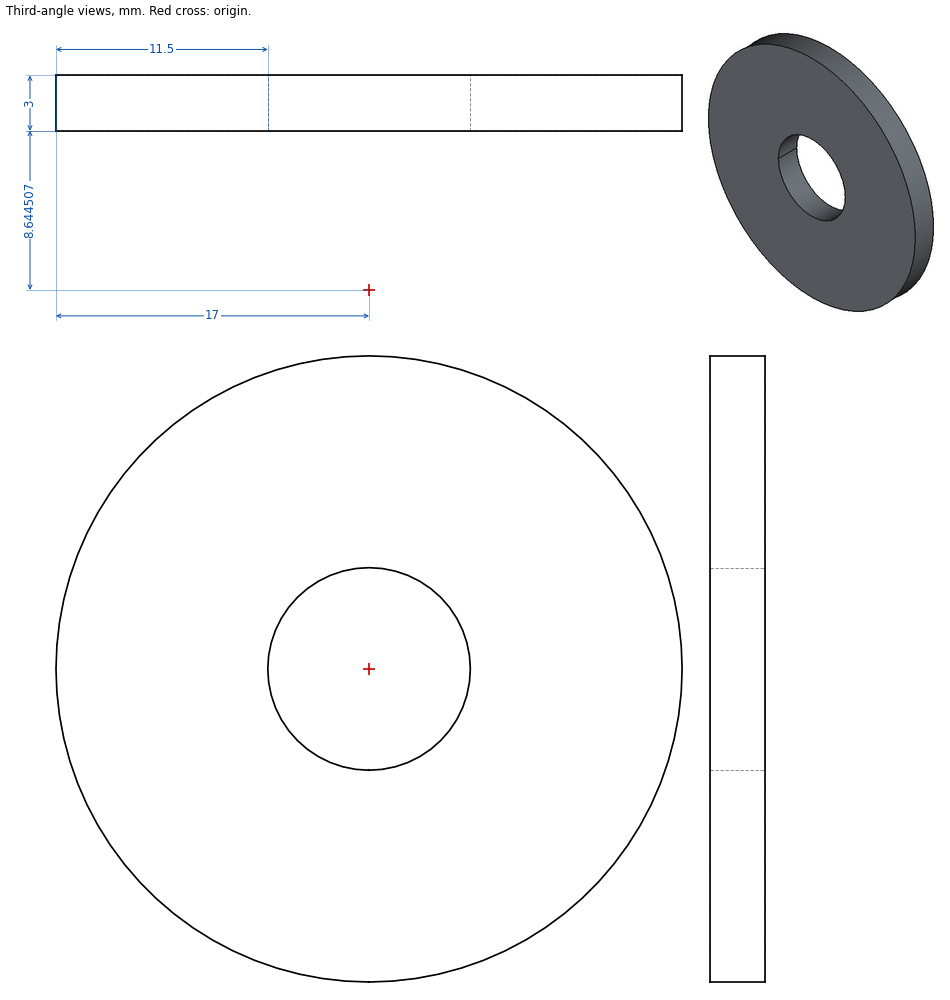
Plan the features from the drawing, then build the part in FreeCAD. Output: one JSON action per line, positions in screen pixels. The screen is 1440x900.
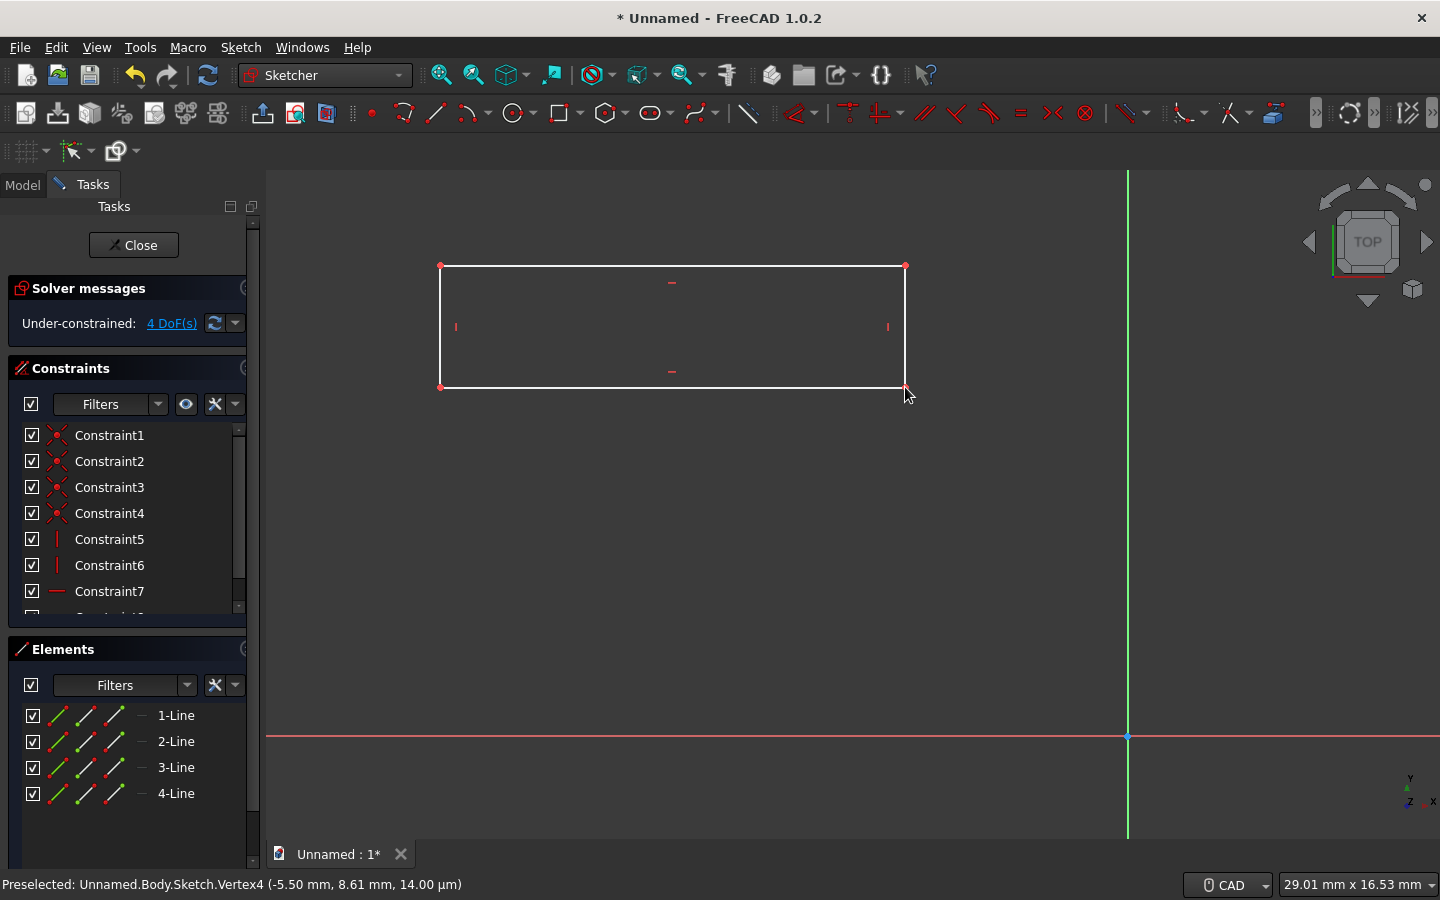
{"action": "left_click", "coordinate": [794, 114]}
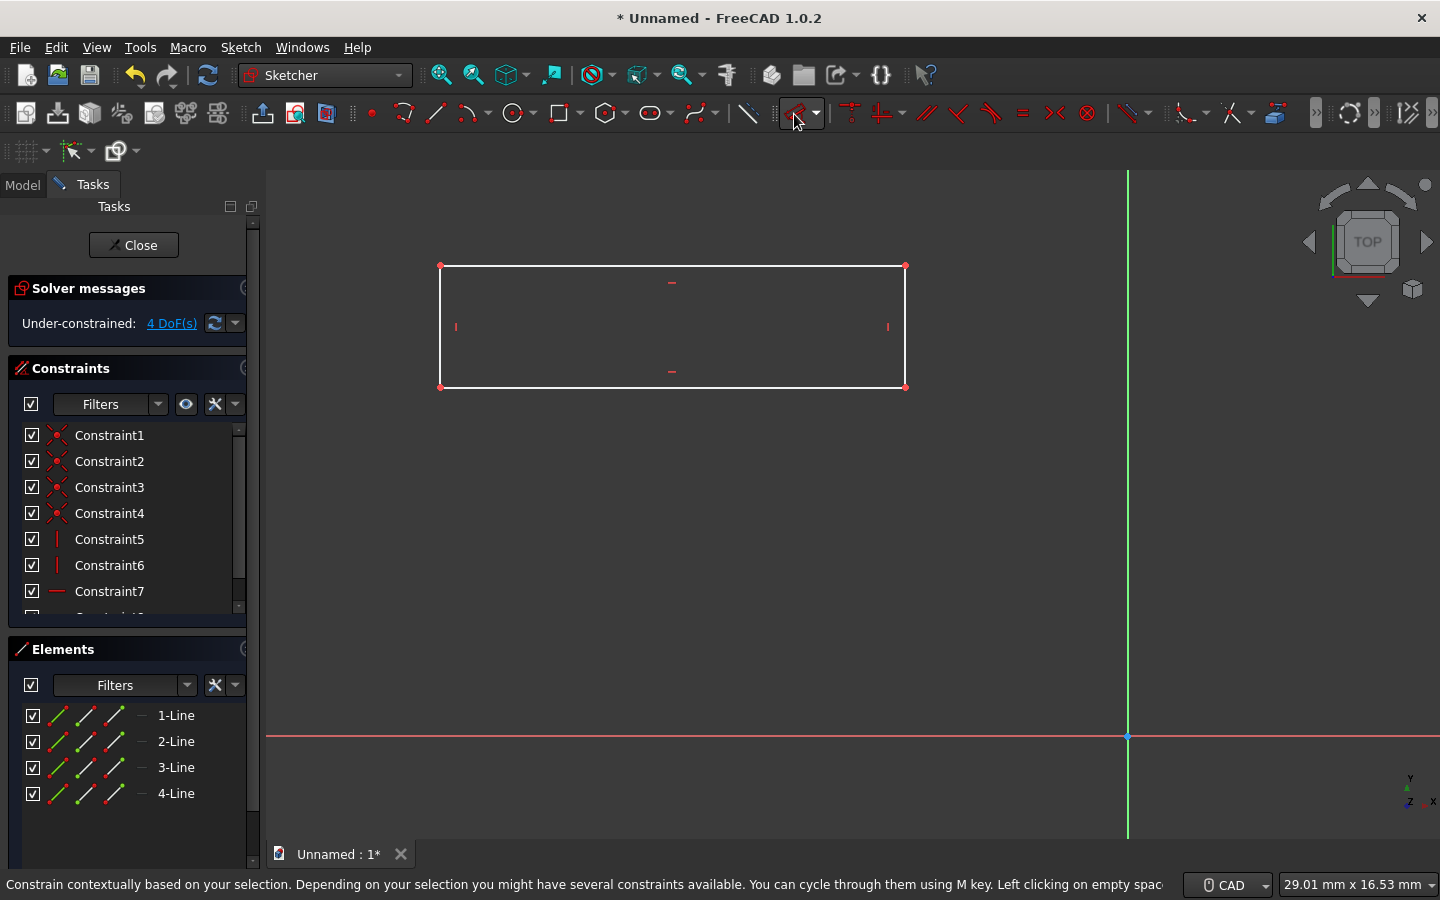
{"action": "left_click", "coordinate": [440, 303]}
{"action": "left_click", "coordinate": [406, 327]}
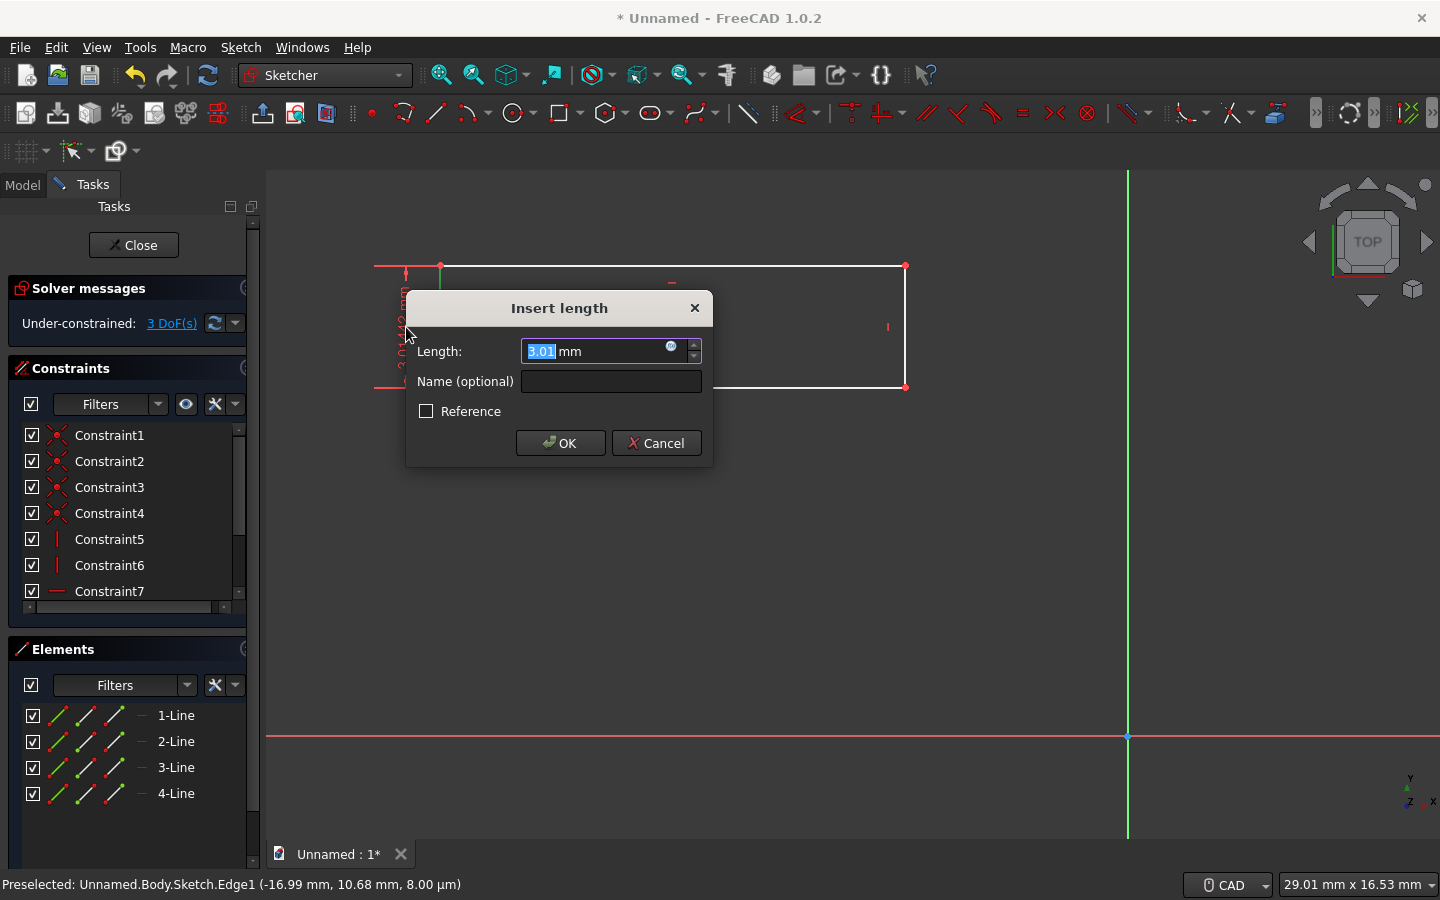
{"action": "type", "text": "3"}
{"action": "key", "text": "Return"}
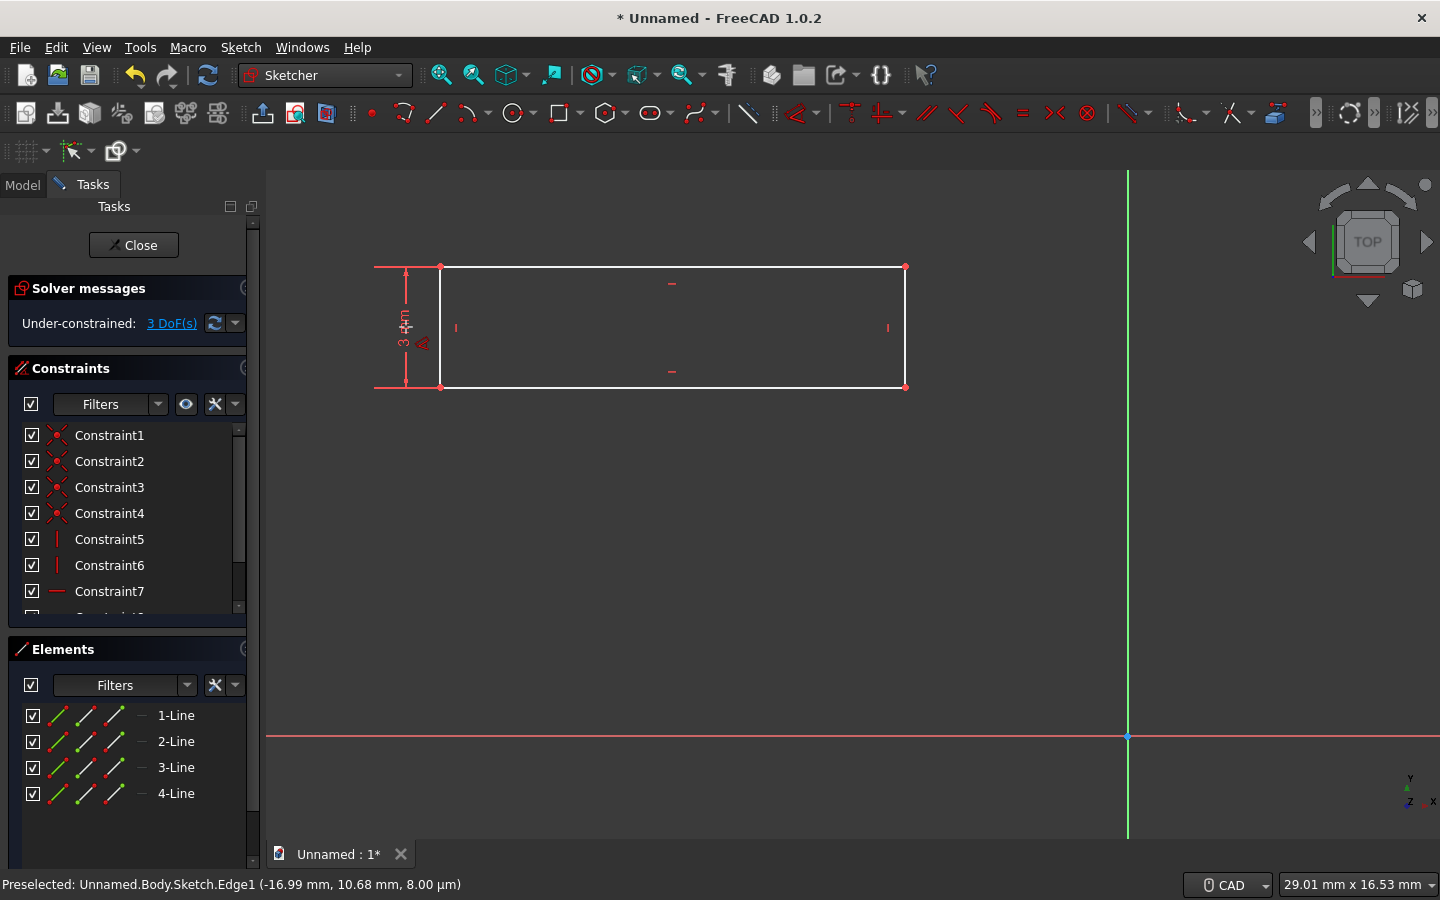
{"action": "left_click", "coordinate": [440, 267]}
{"action": "left_click", "coordinate": [784, 770]}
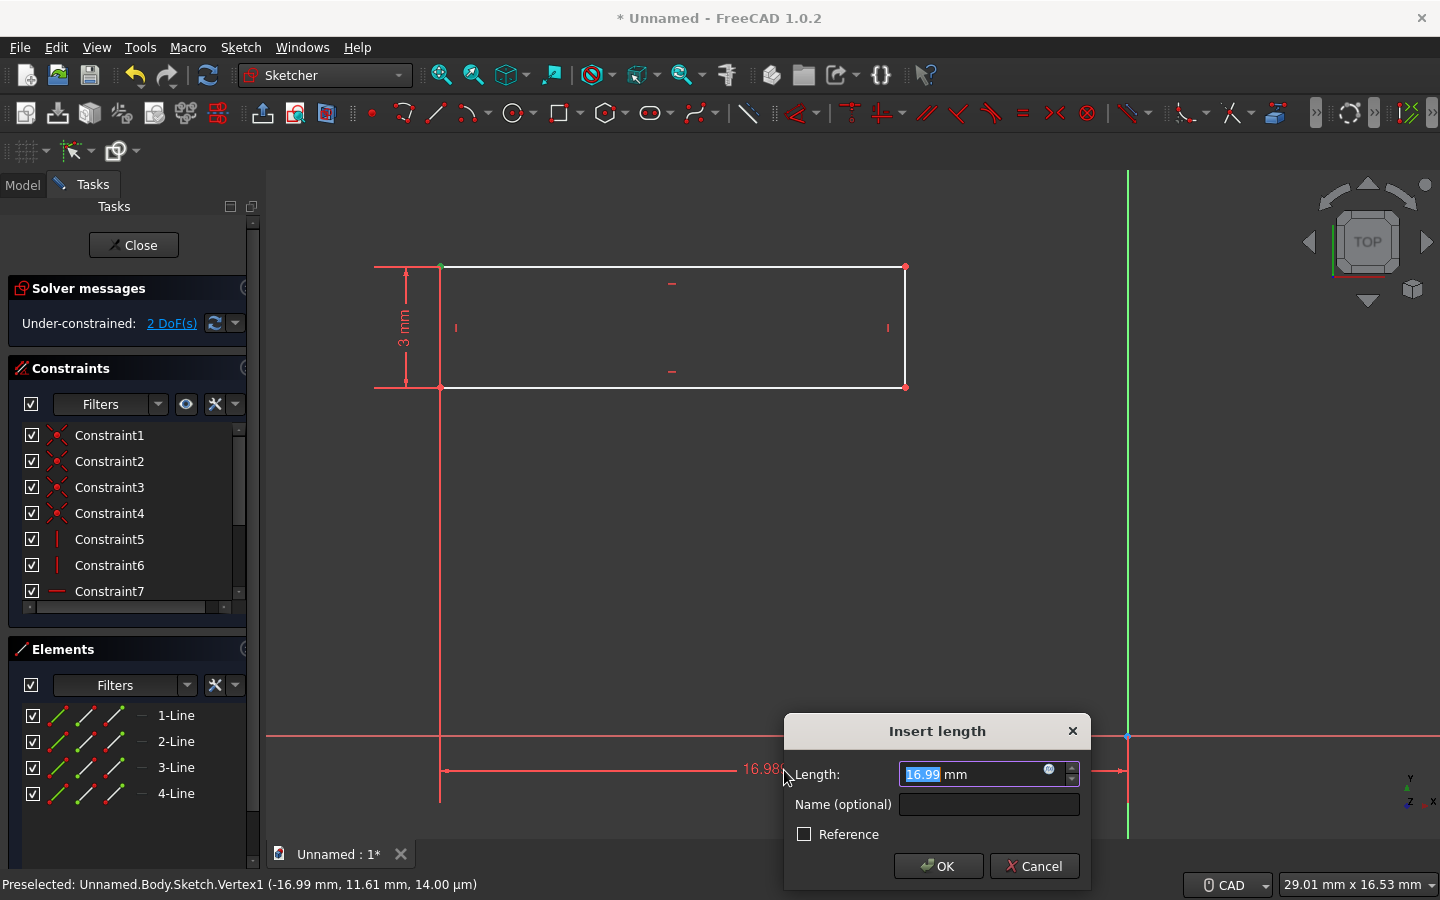
{"action": "type", "text": "17"}
{"action": "key", "text": "Return"}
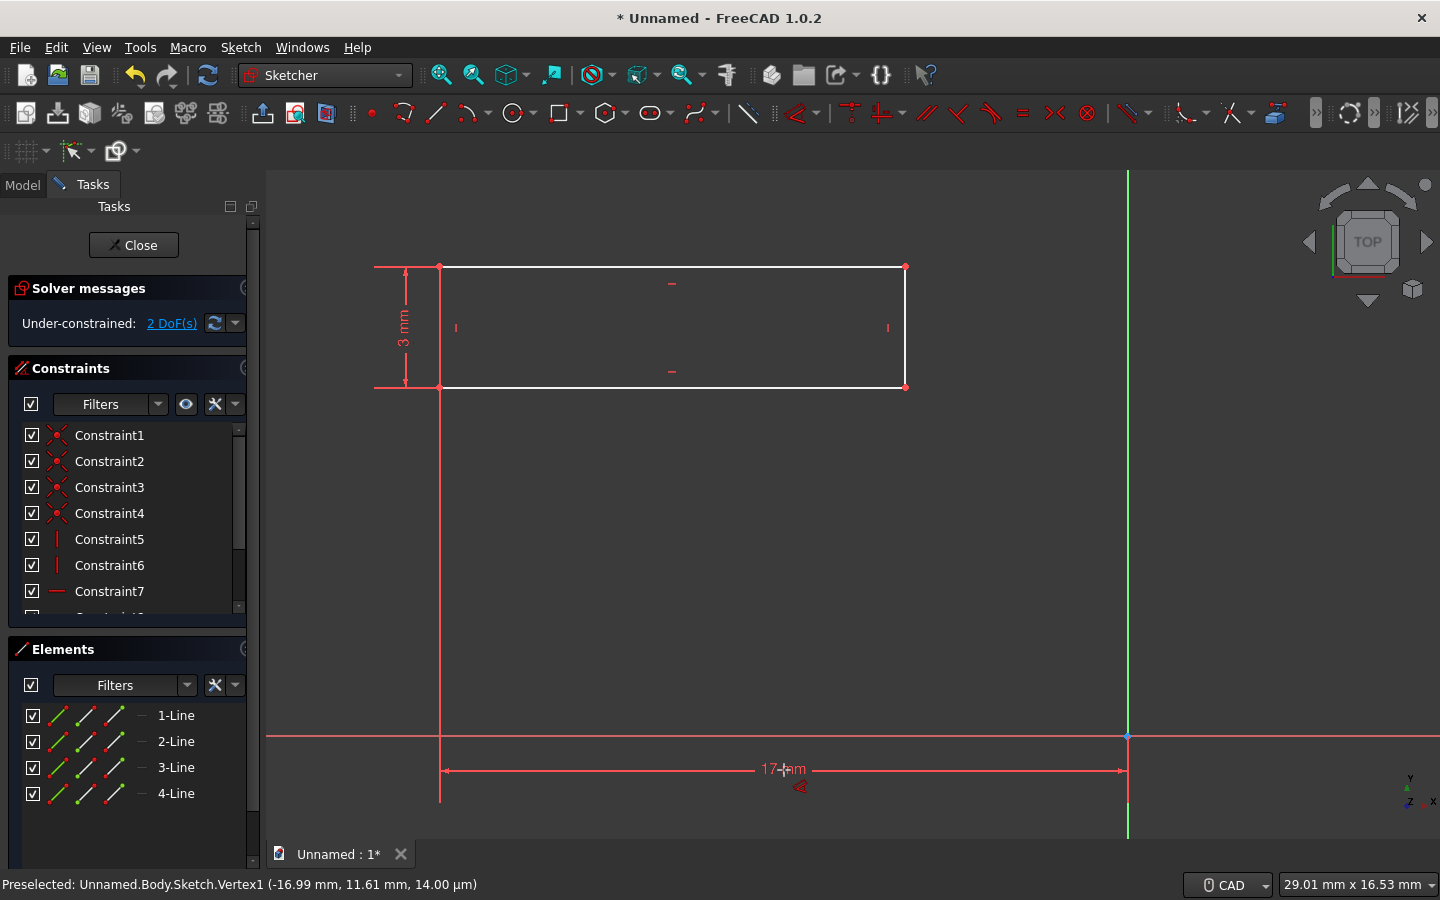
{"action": "left_click", "coordinate": [579, 388]}
{"action": "left_click", "coordinate": [672, 354]}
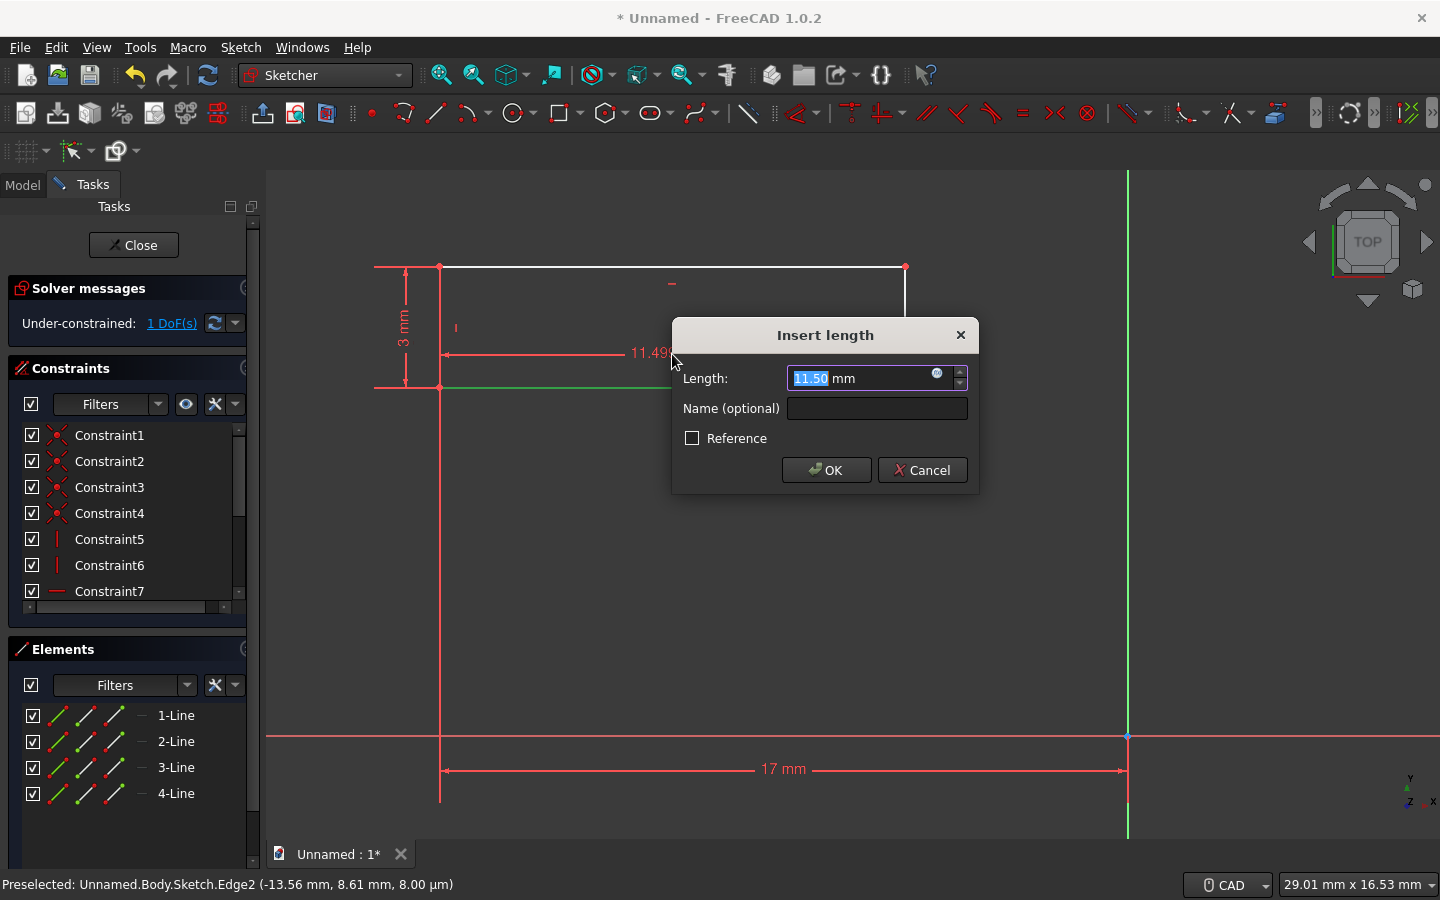
{"action": "type", "text": "11.5"}
{"action": "key", "text": "Return"}